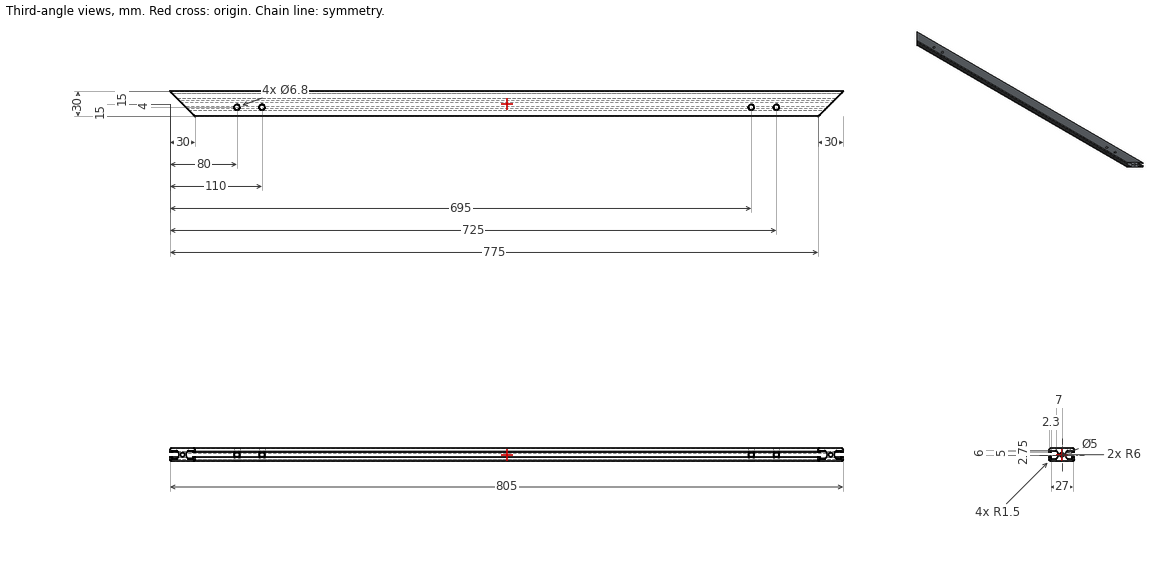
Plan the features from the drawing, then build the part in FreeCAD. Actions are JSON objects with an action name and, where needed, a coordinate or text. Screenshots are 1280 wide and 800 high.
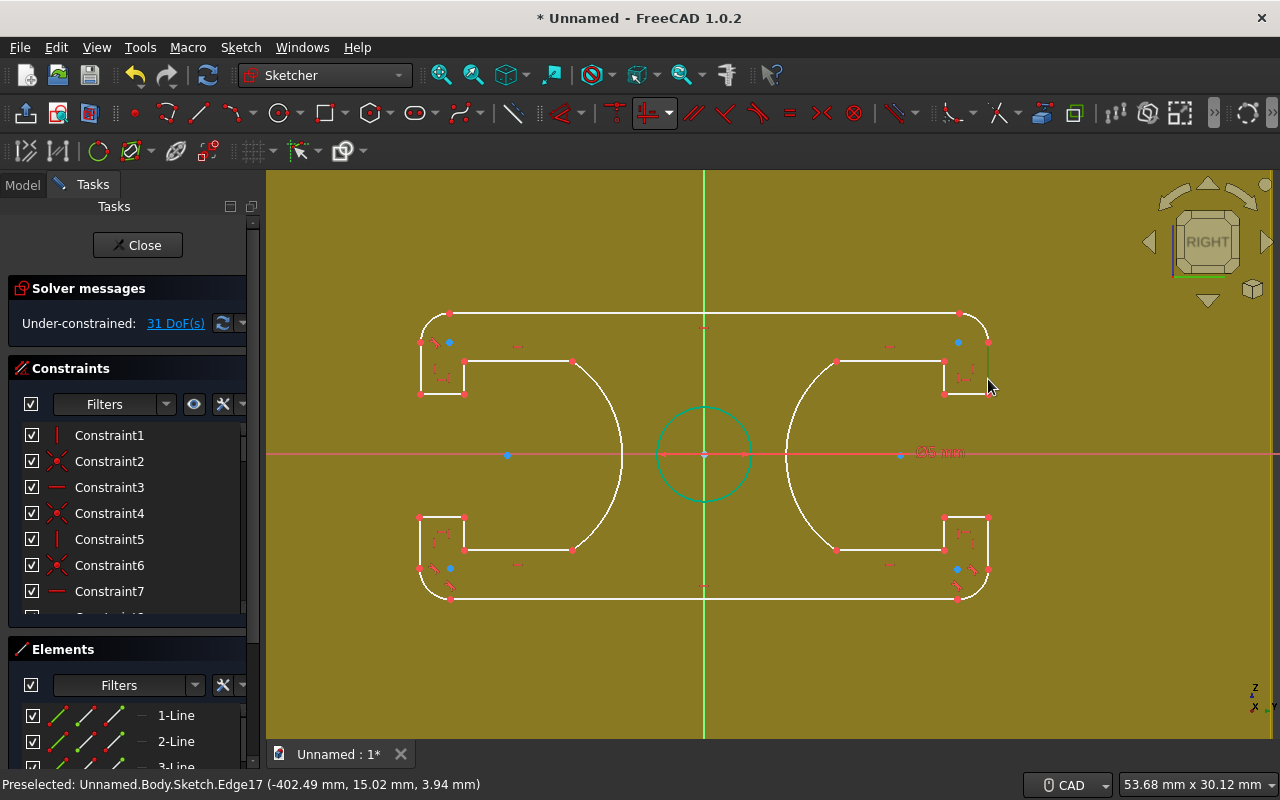
{"action": "left_click", "coordinate": [985, 329]}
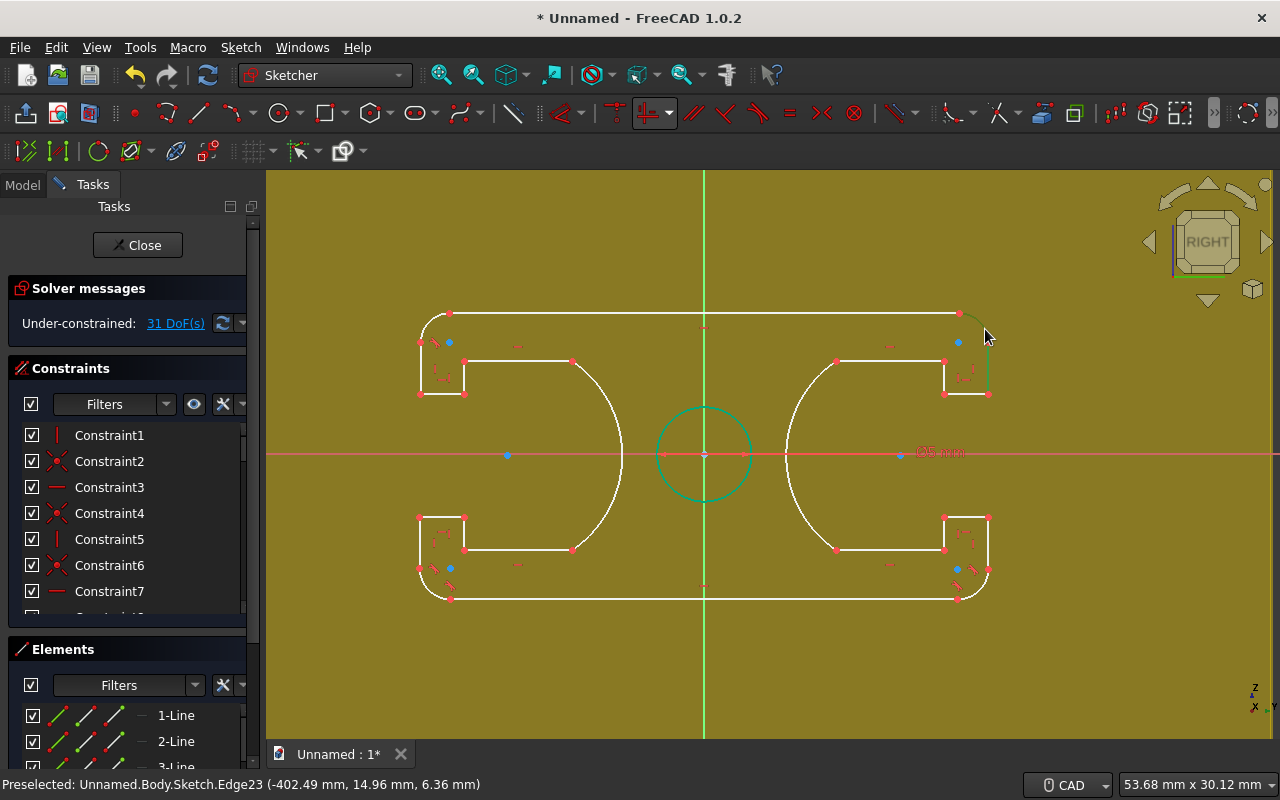
{"action": "left_click", "coordinate": [758, 114]}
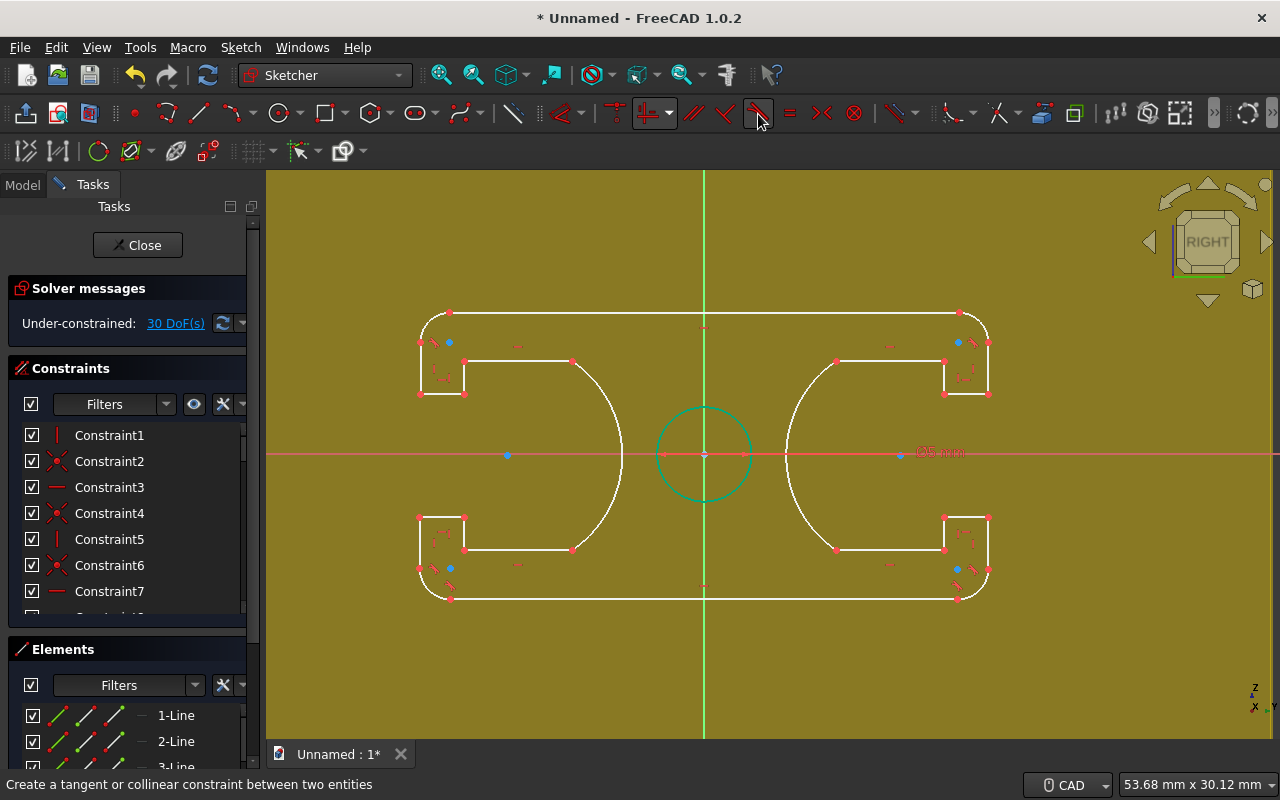
{"action": "left_click", "coordinate": [806, 313]}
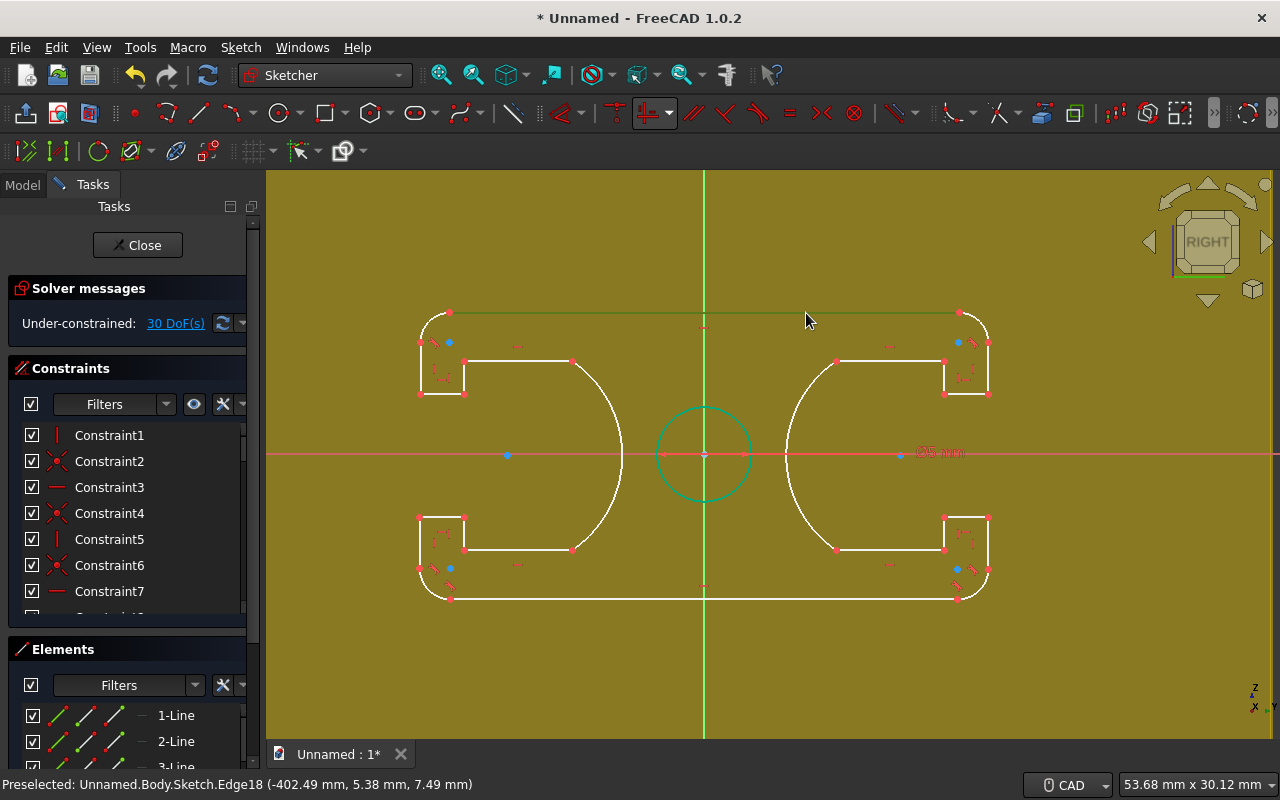
{"action": "left_click", "coordinate": [985, 329]}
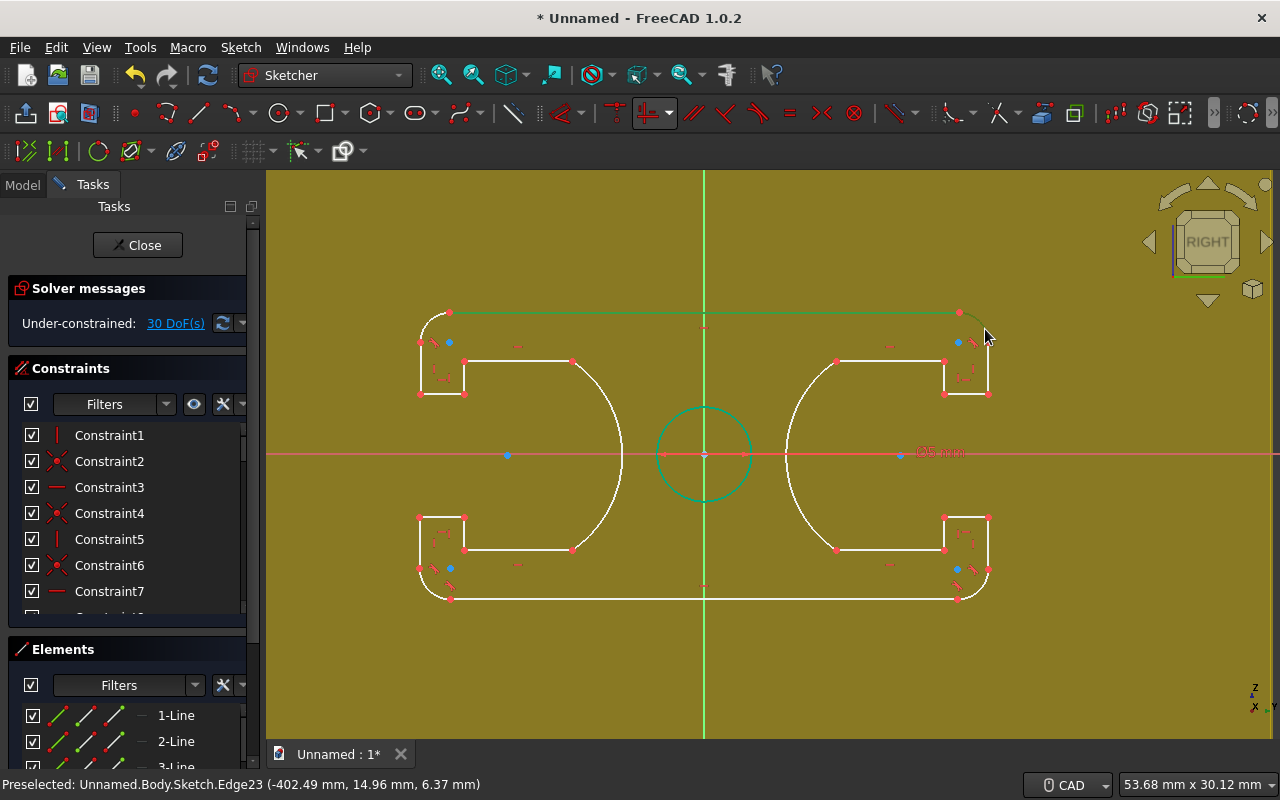
{"action": "left_click", "coordinate": [758, 114]}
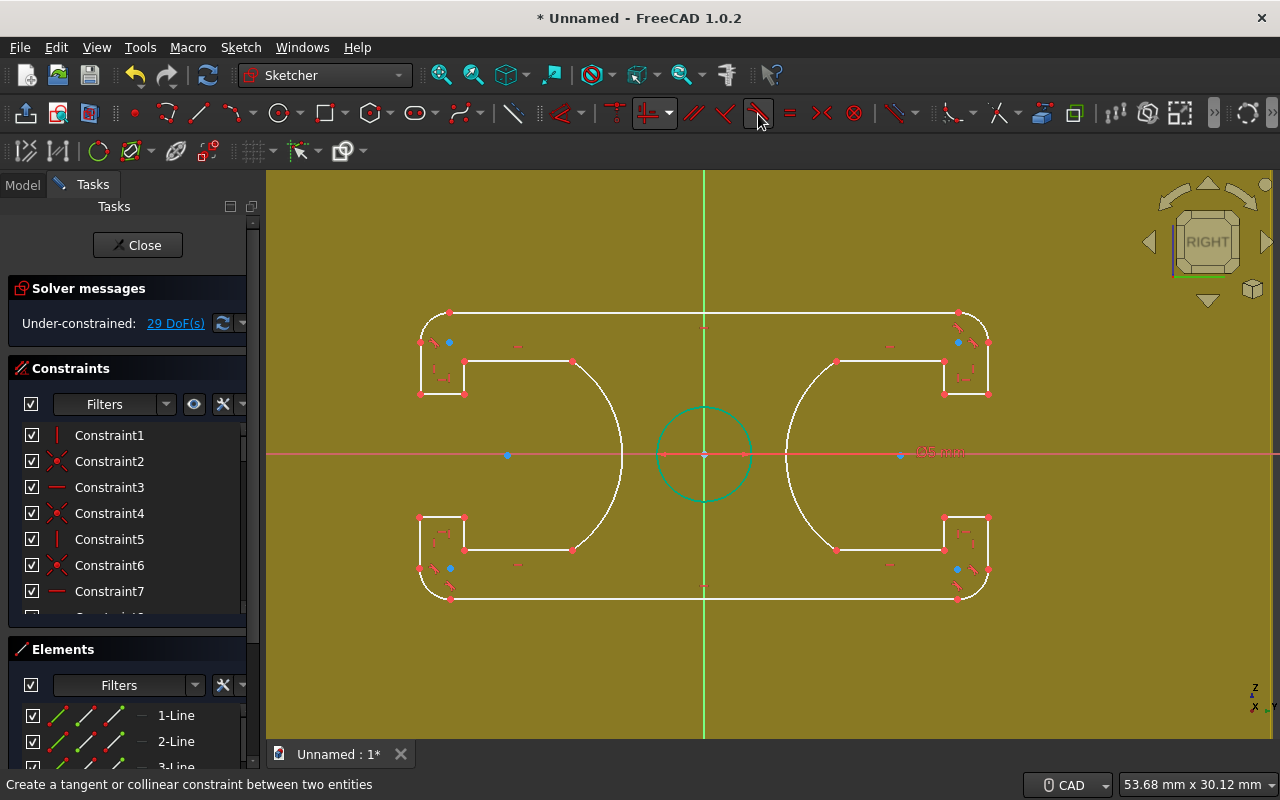
{"action": "left_click", "coordinate": [806, 313]}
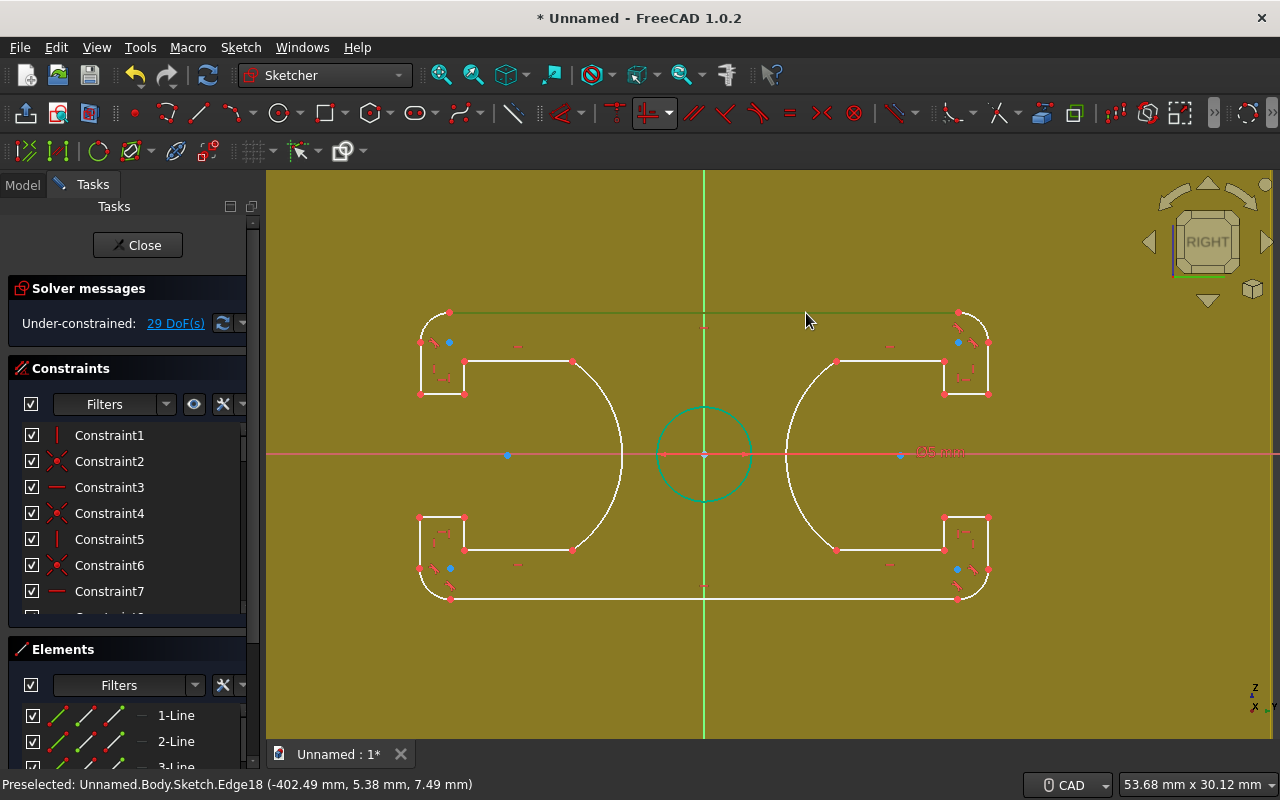
{"action": "left_click", "coordinate": [436, 316]}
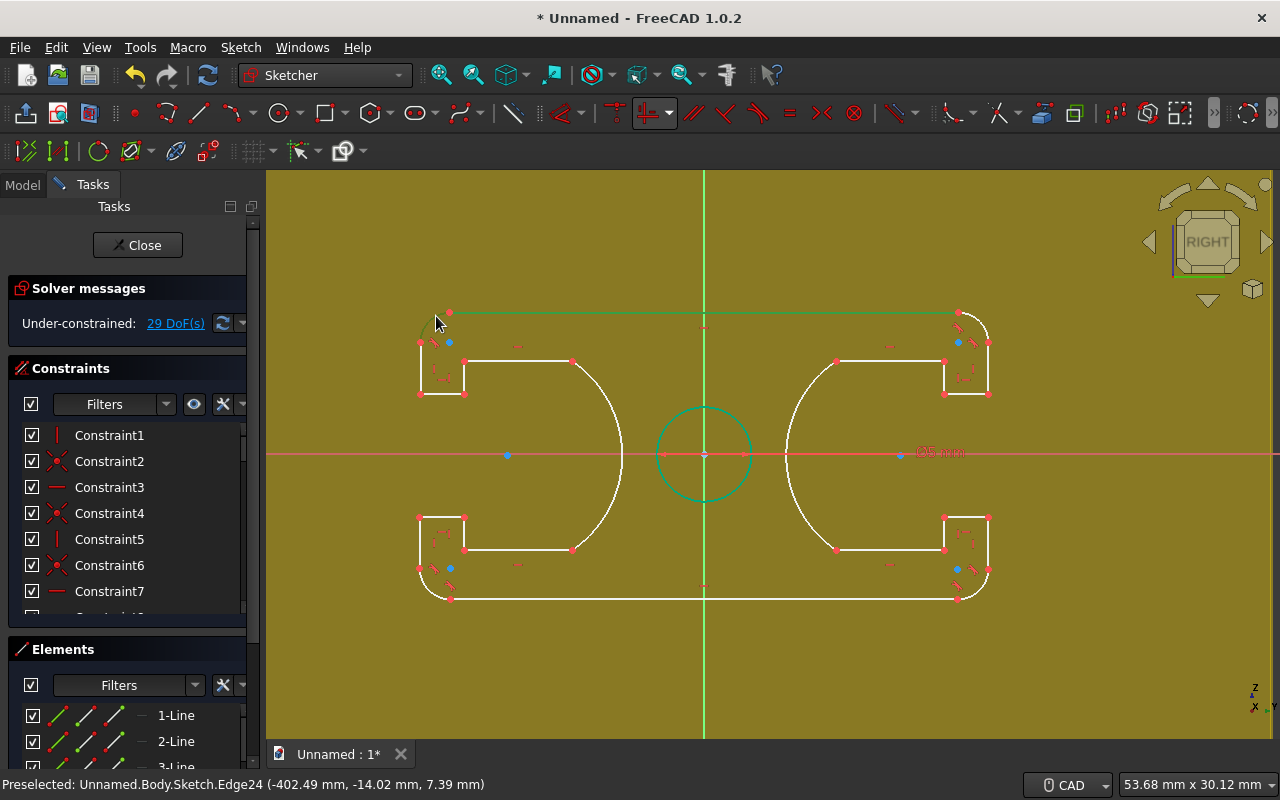
{"action": "left_click", "coordinate": [758, 114]}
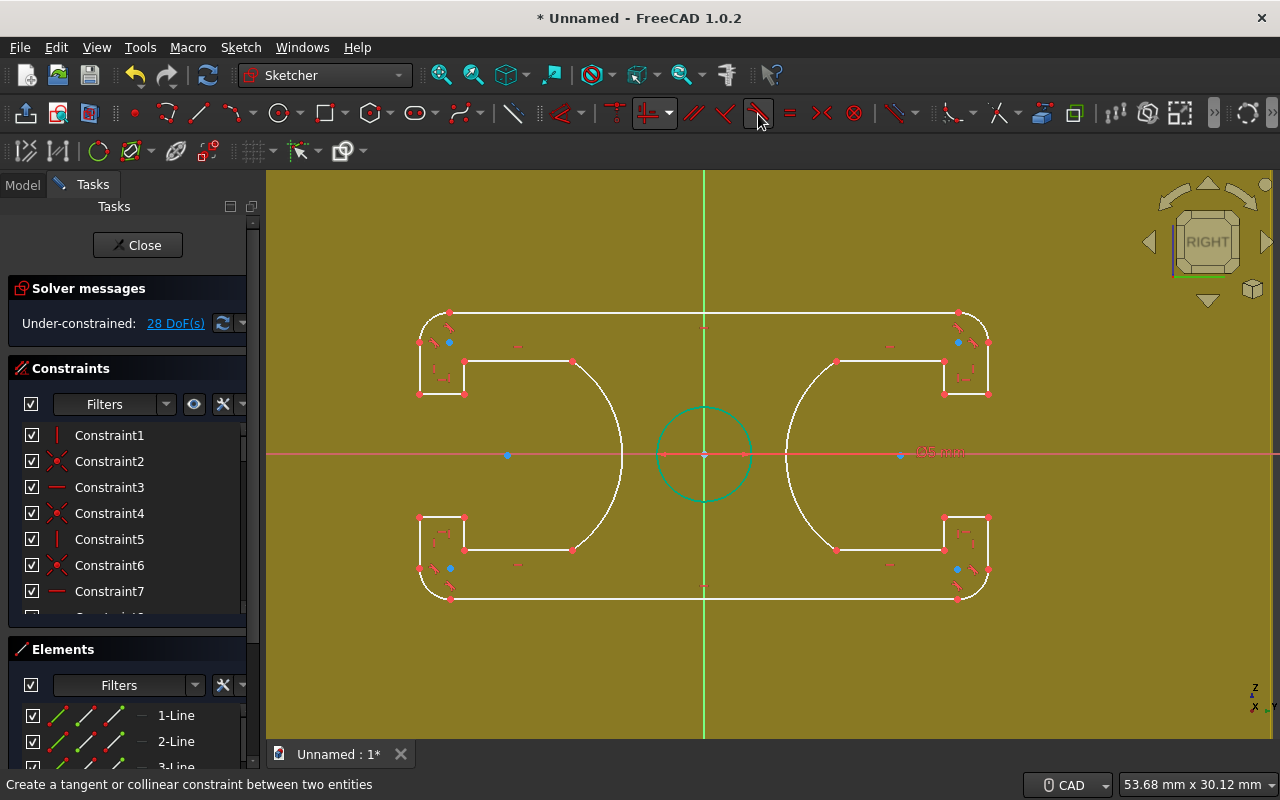
{"action": "left_click", "coordinate": [423, 583]}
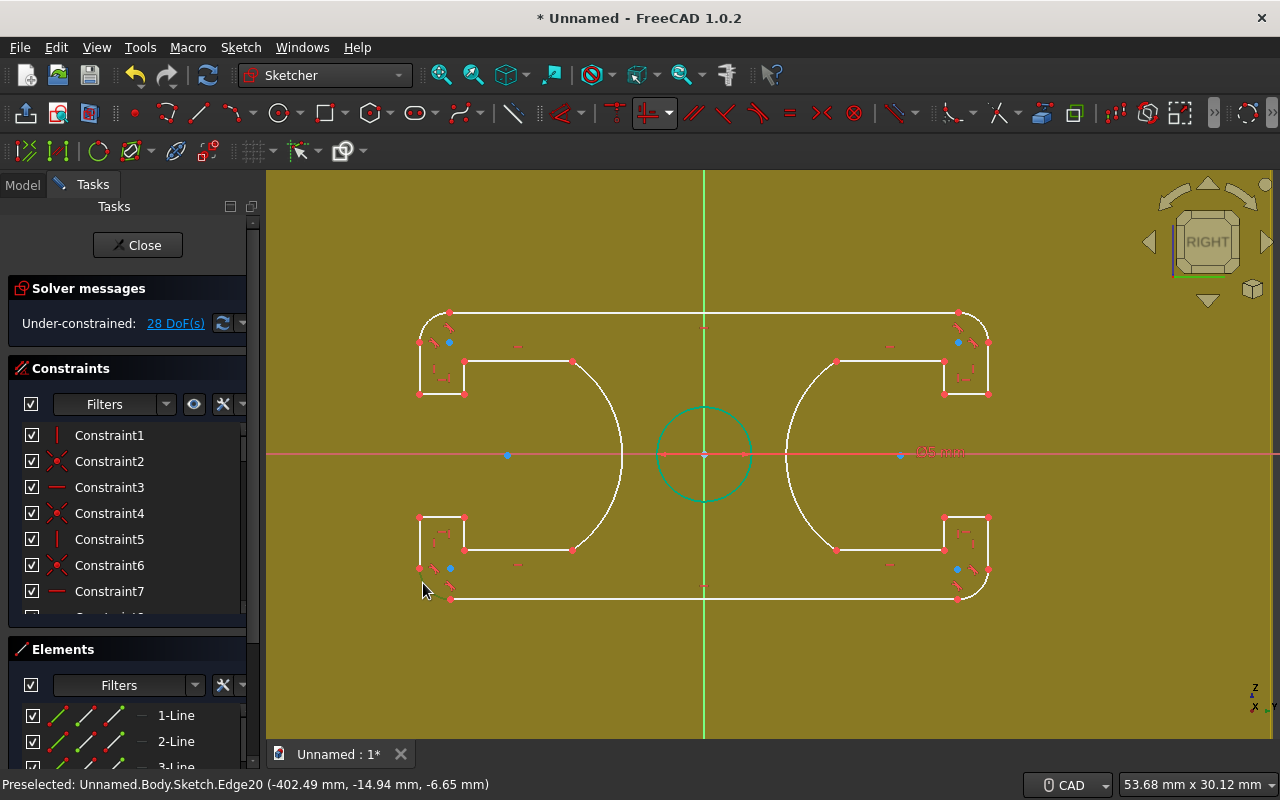
{"action": "left_click", "coordinate": [972, 596]}